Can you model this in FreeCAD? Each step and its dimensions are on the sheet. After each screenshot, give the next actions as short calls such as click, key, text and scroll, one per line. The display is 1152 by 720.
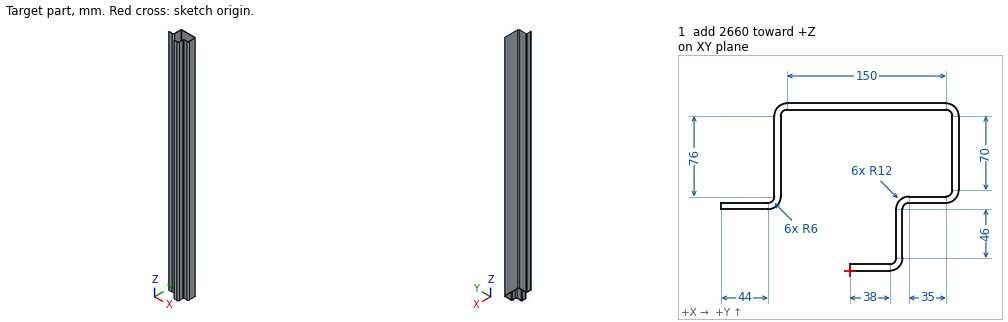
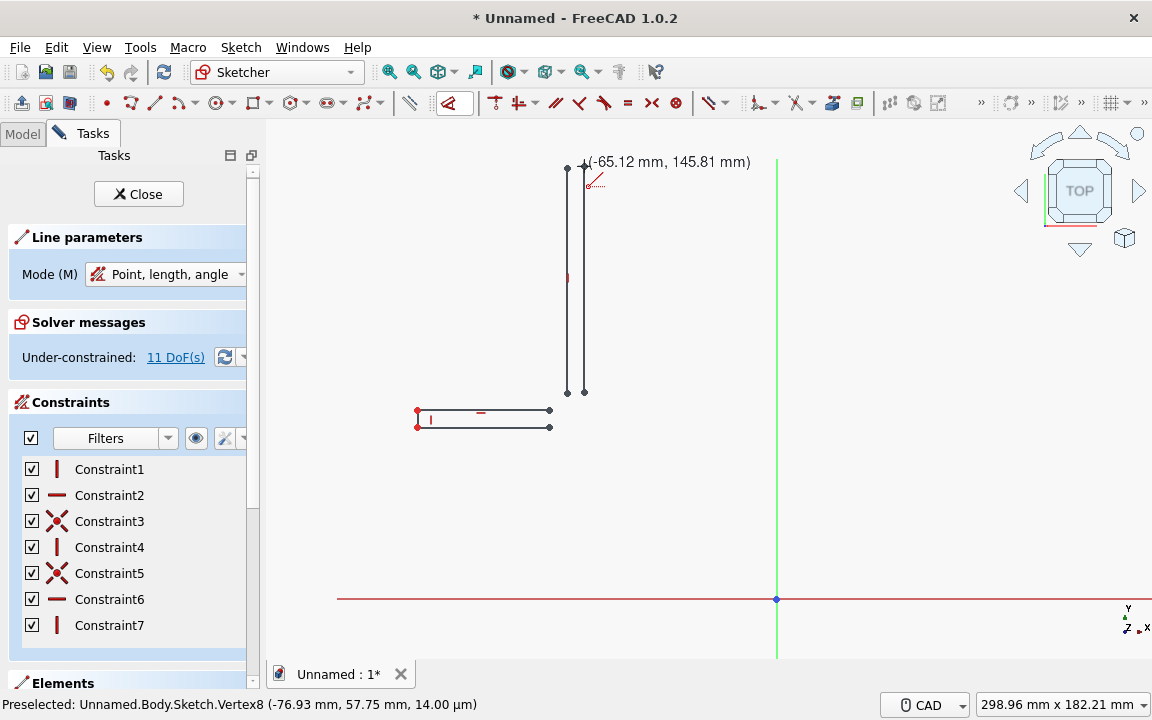
click(602, 149)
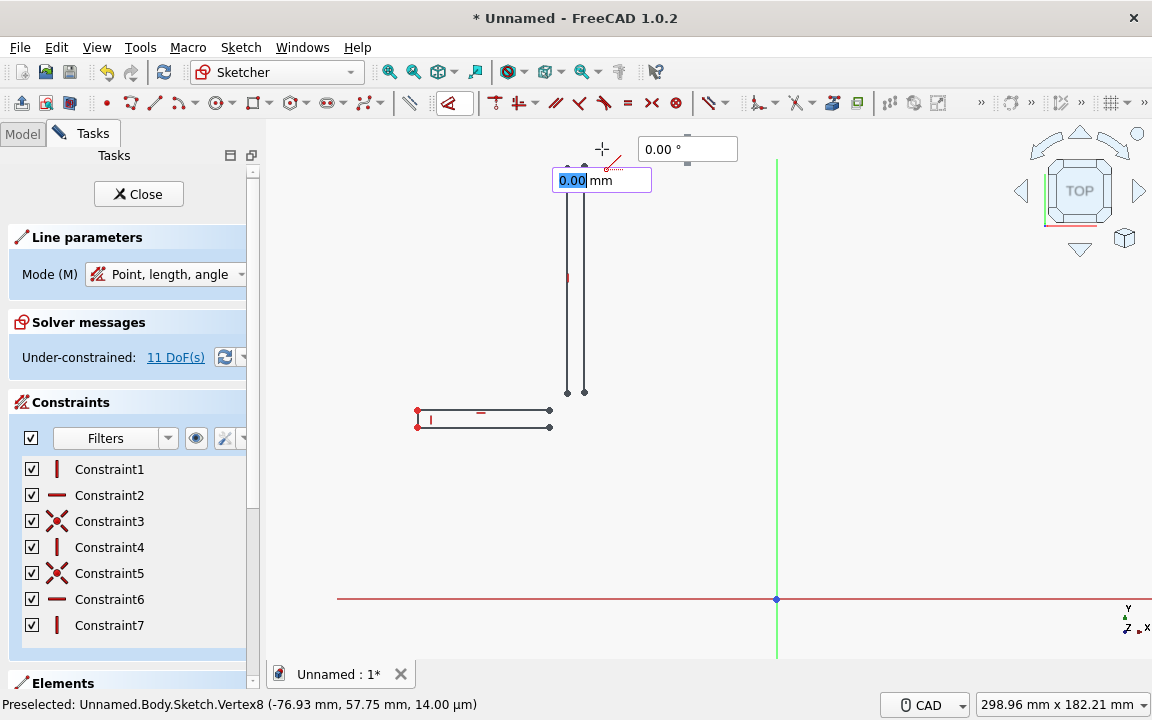
scroll(417, 438, down, 2)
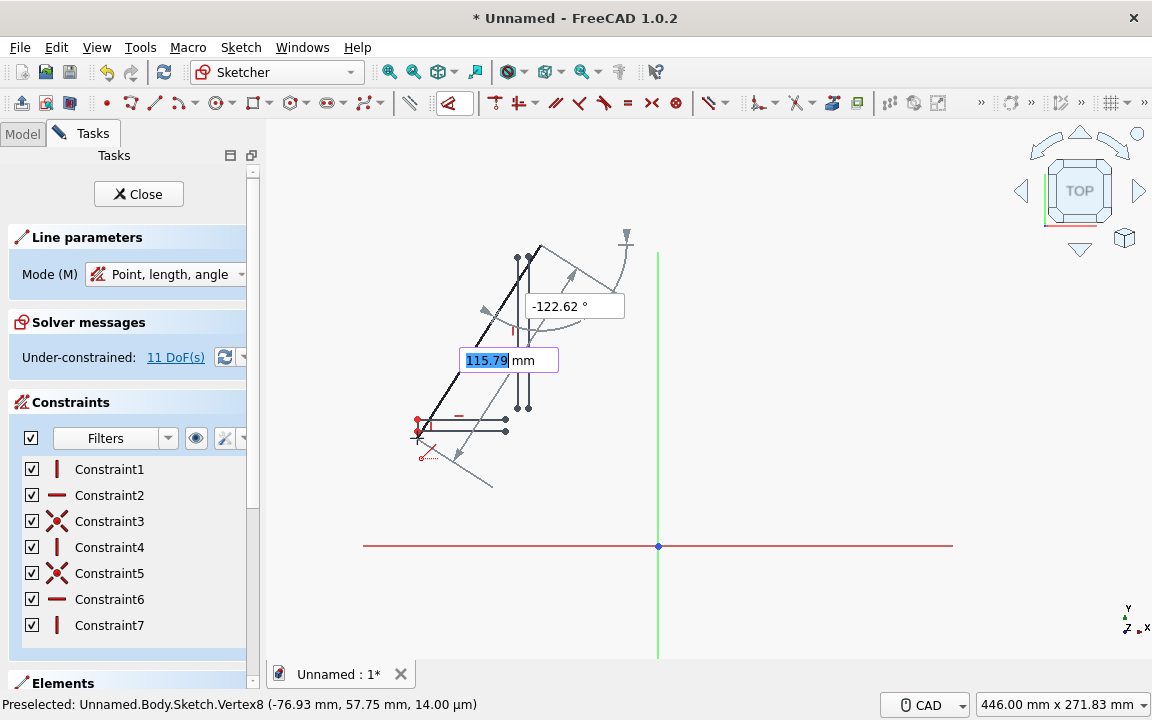
click(839, 244)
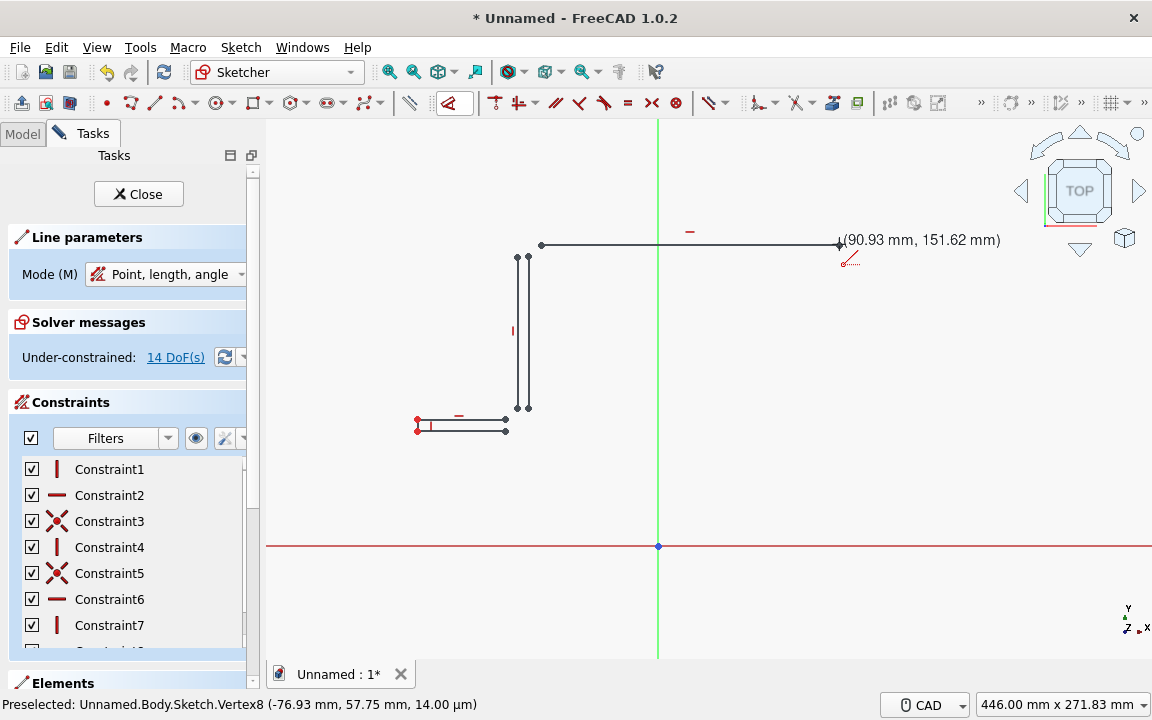
click(851, 256)
click(851, 395)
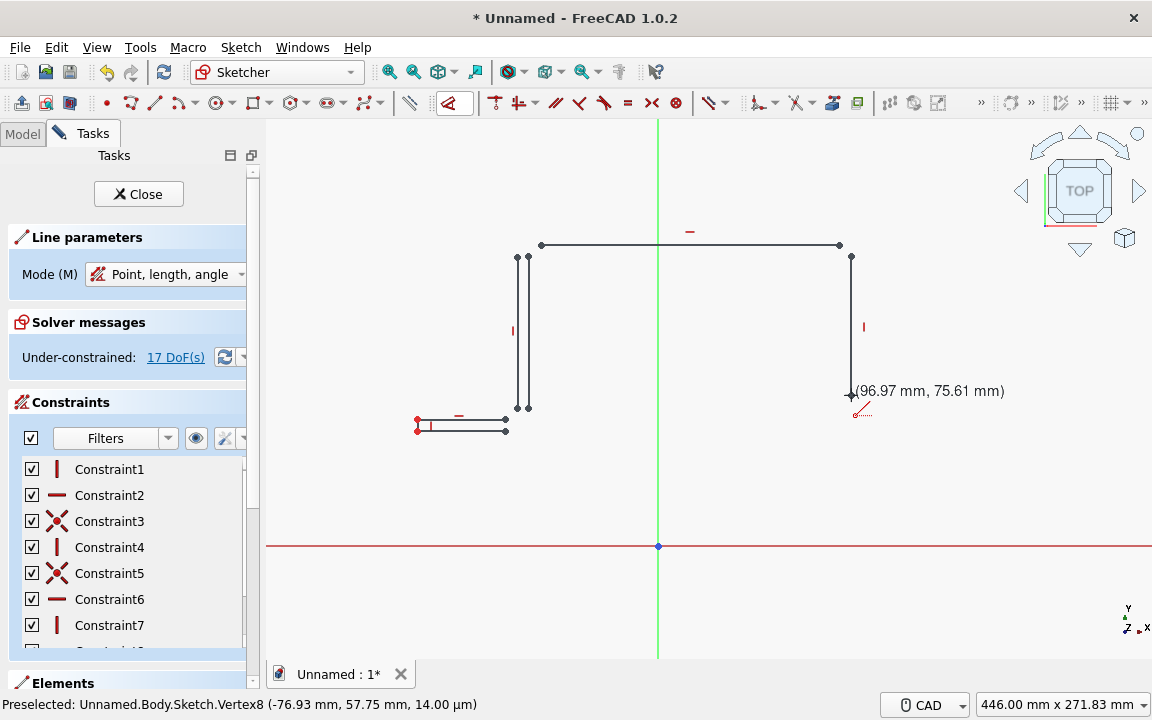
click(839, 407)
click(770, 407)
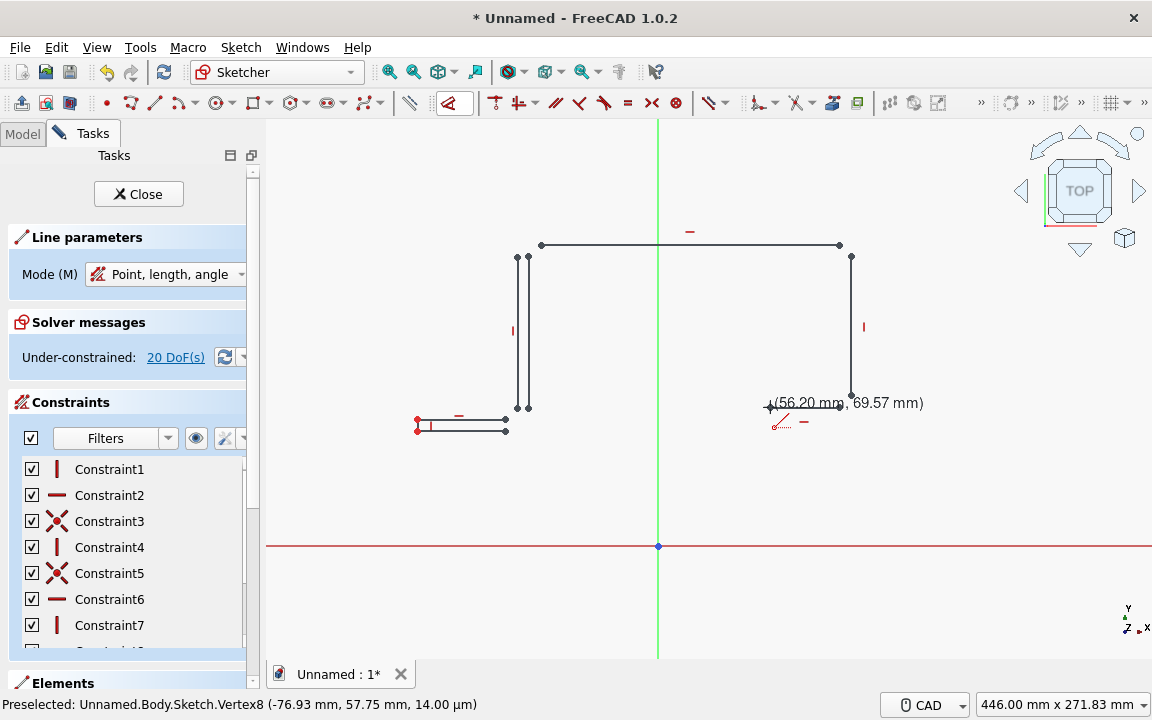
click(746, 431)
click(746, 522)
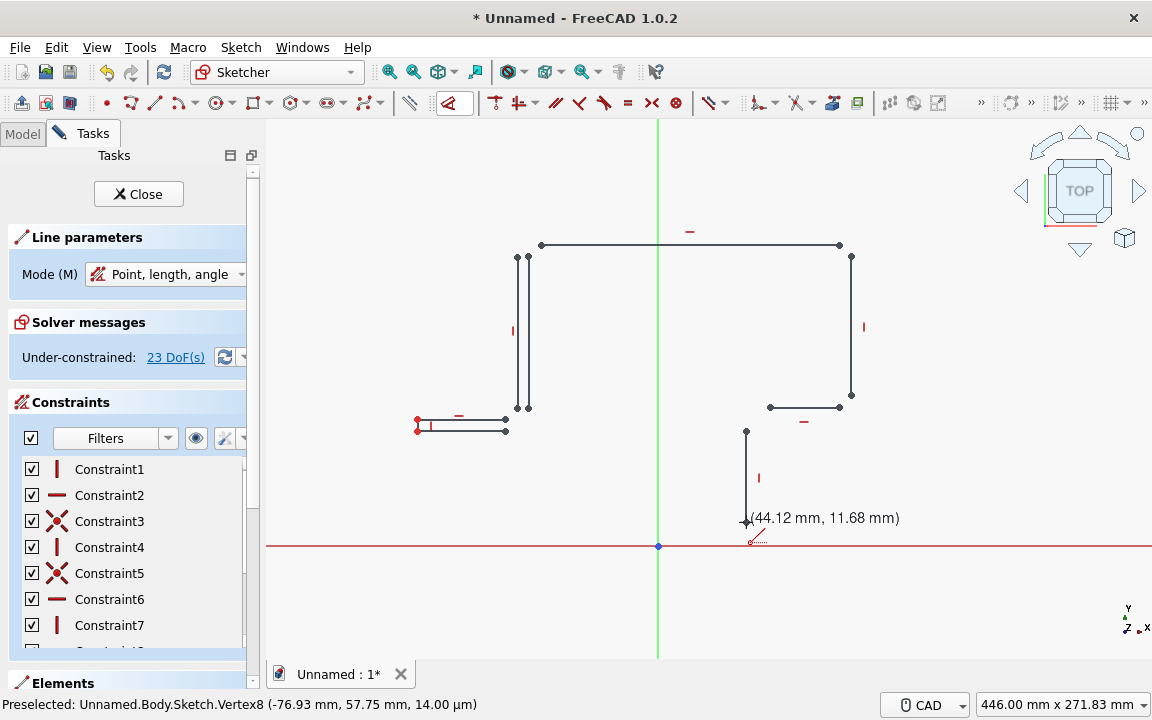
key(g)
key(m)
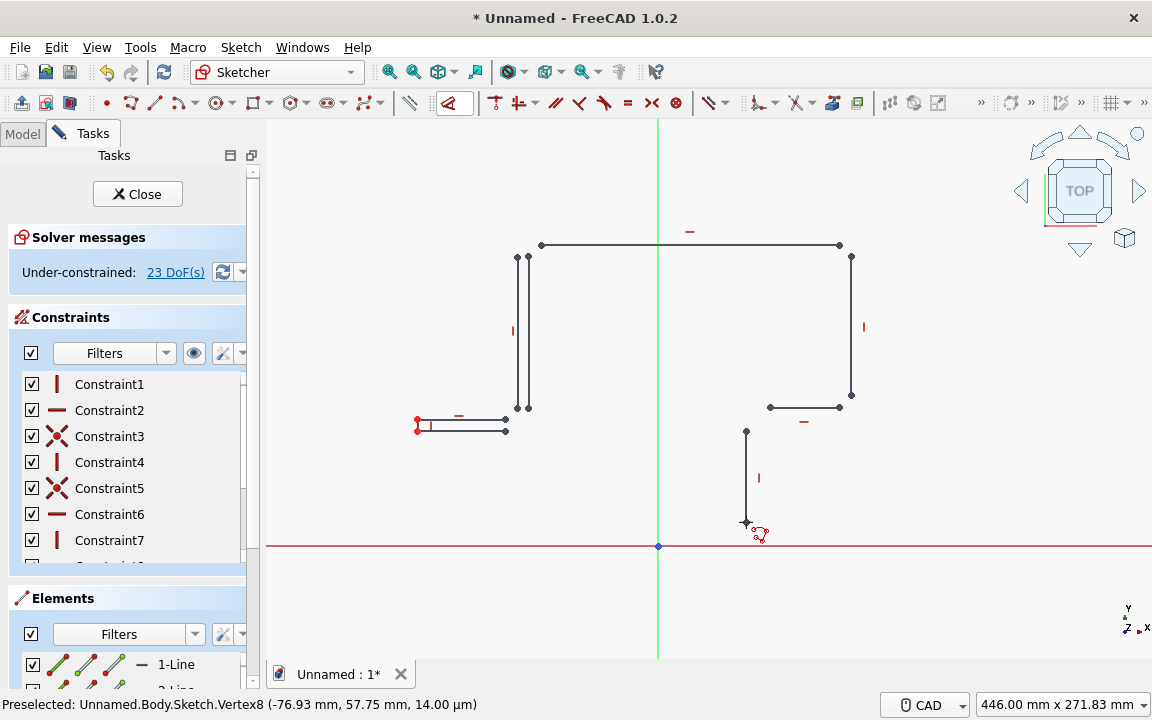
scroll(734, 534, up, 2)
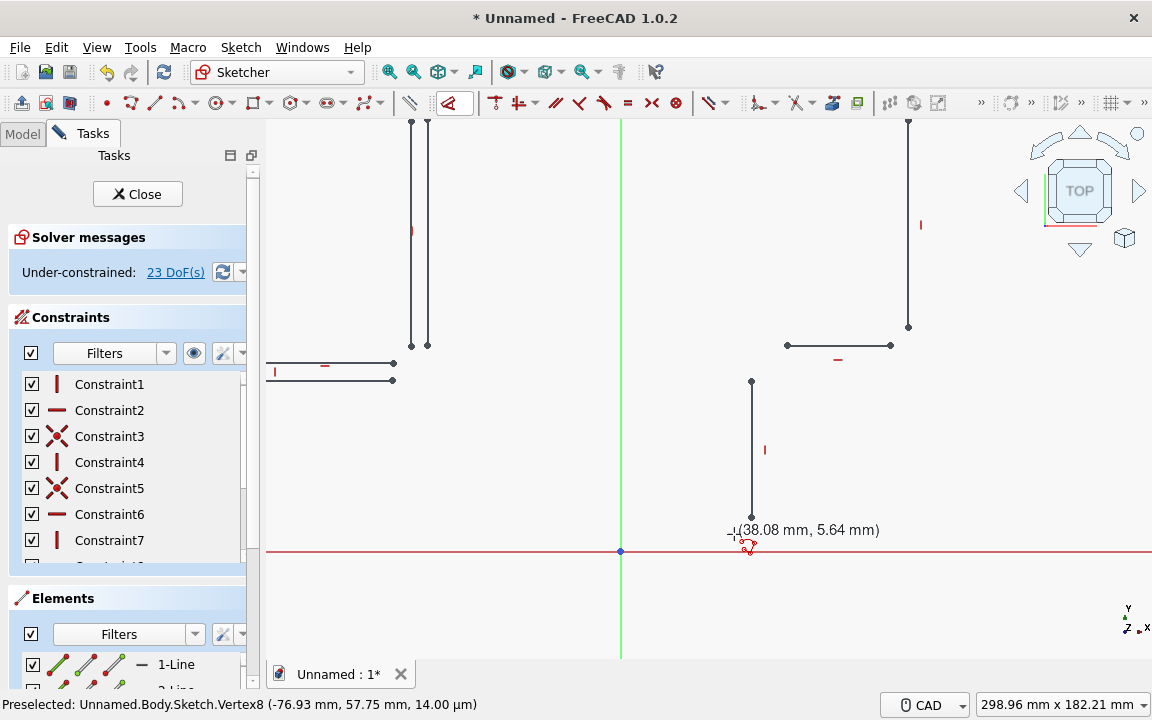
click(734, 534)
click(621, 534)
click(621, 552)
click(734, 543)
right_click(734, 543)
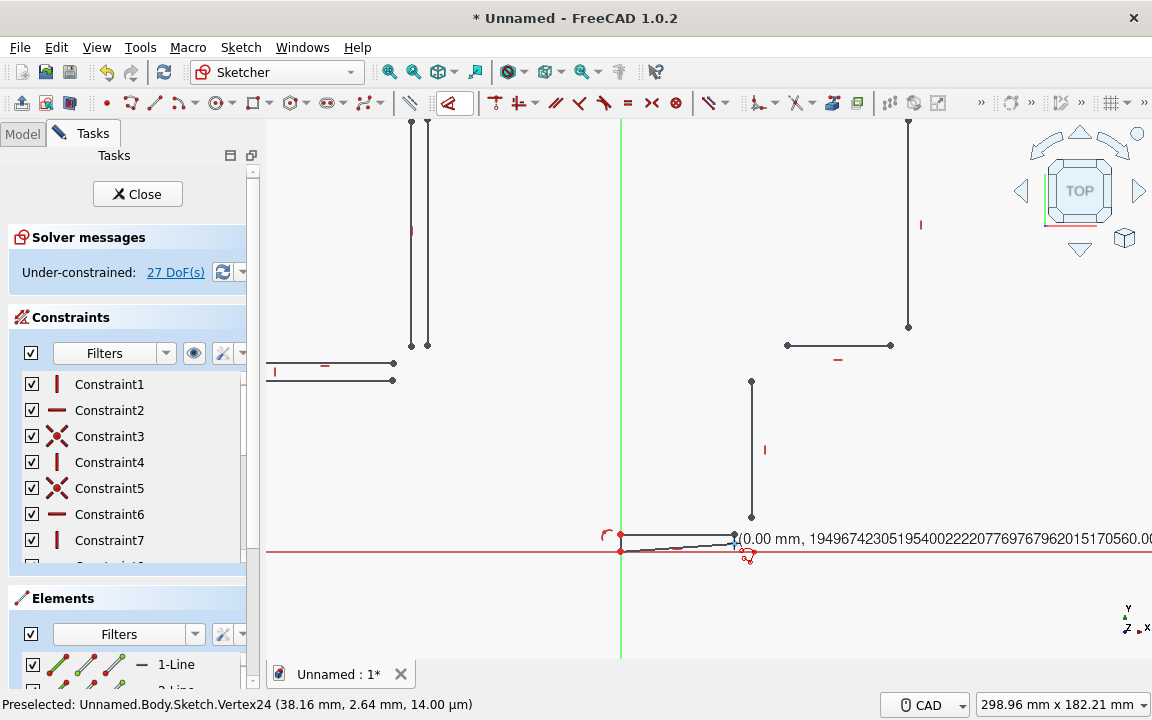
key(g)
key(l)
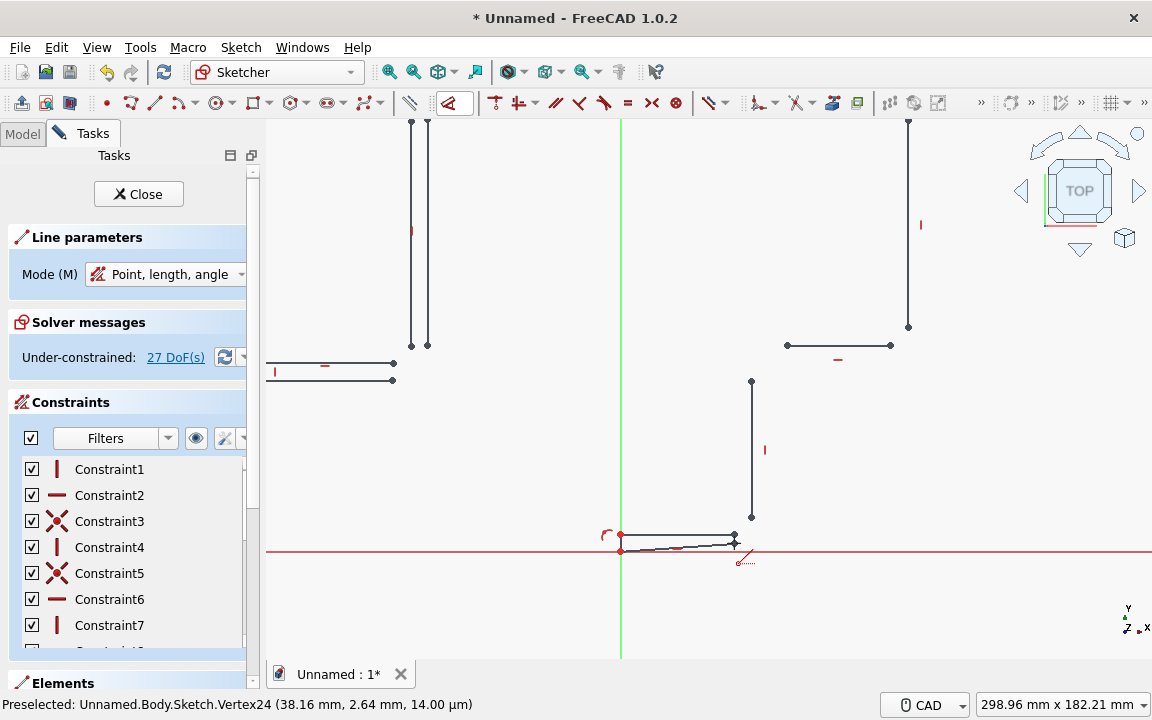
click(769, 516)
click(769, 380)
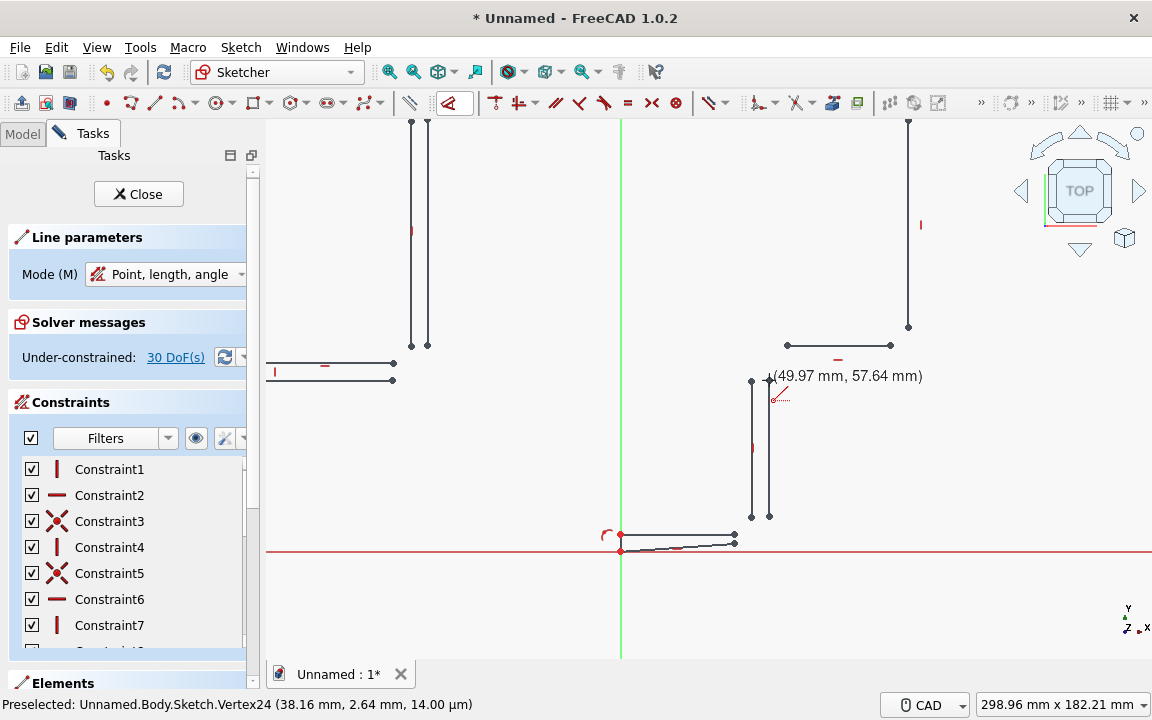
click(787, 362)
click(891, 362)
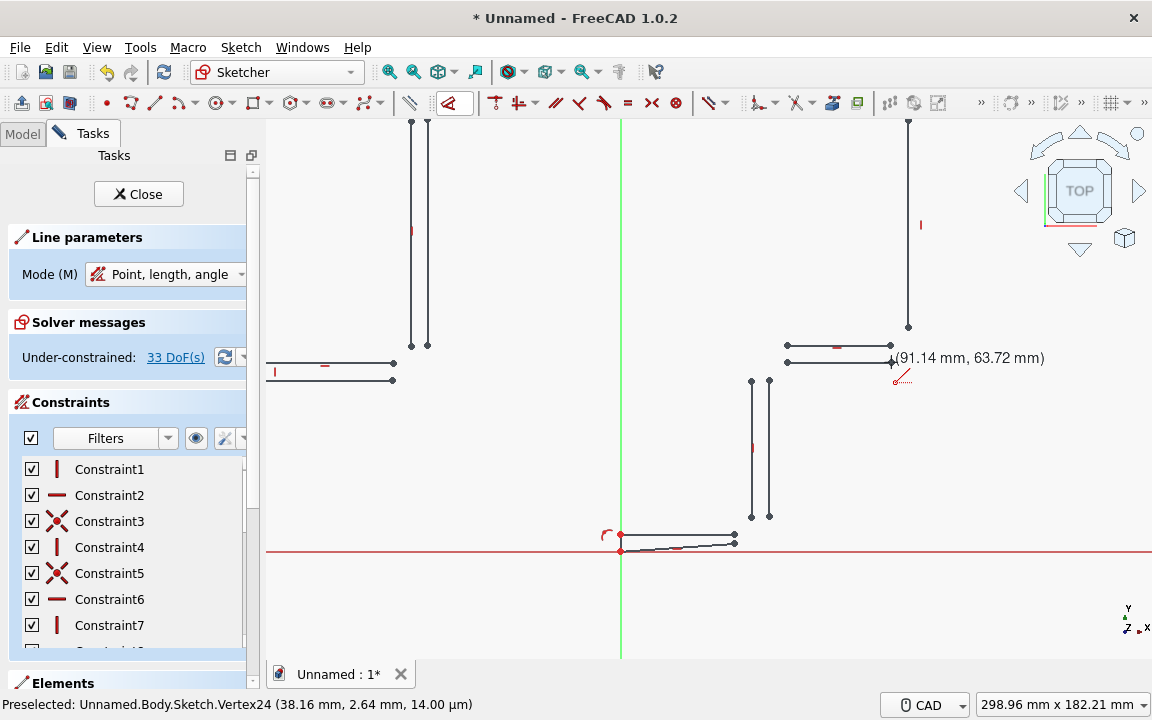
click(926, 327)